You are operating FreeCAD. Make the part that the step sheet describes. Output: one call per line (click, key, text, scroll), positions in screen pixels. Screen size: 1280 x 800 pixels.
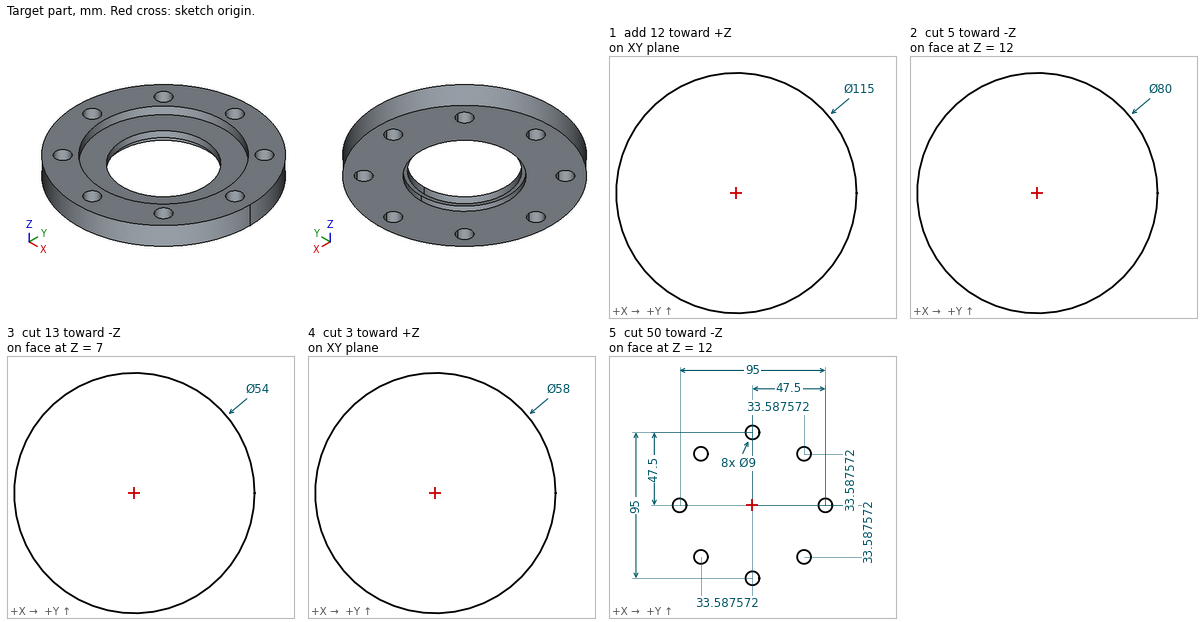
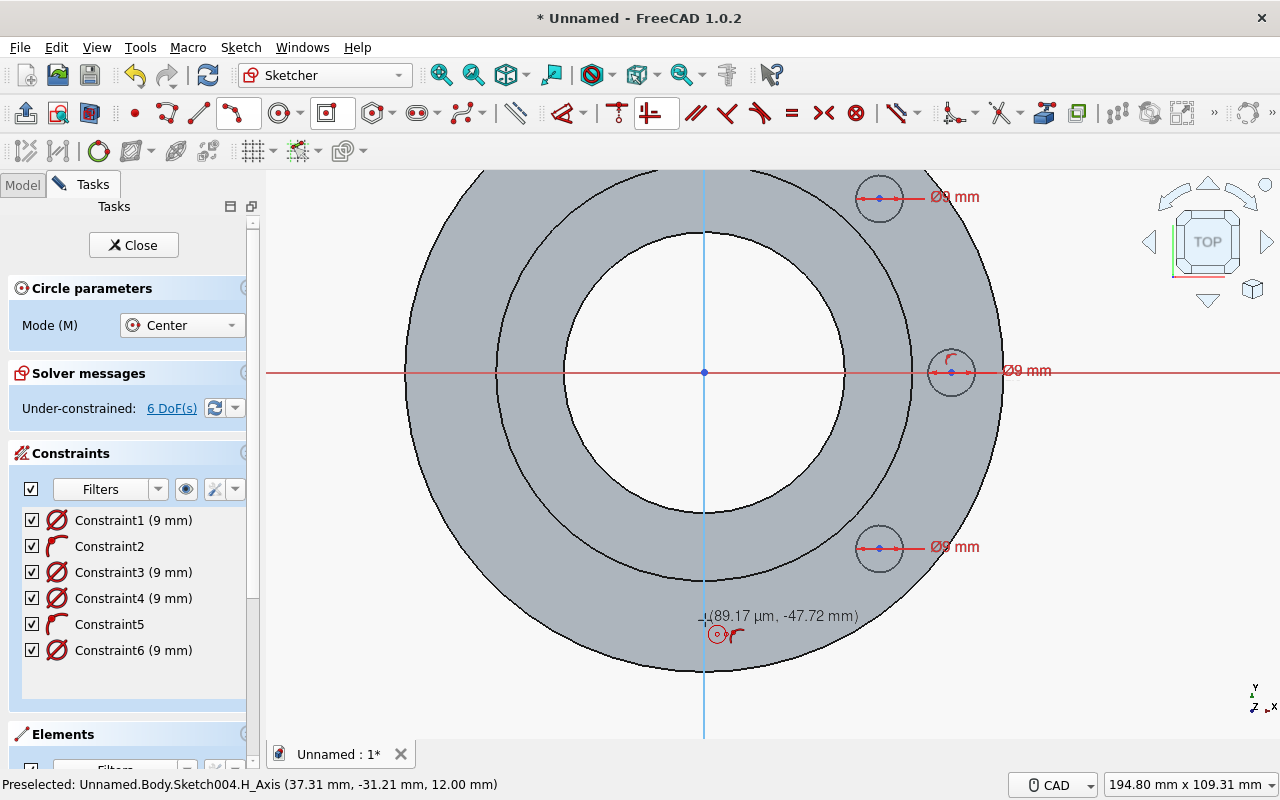
click(704, 620)
move(721, 603)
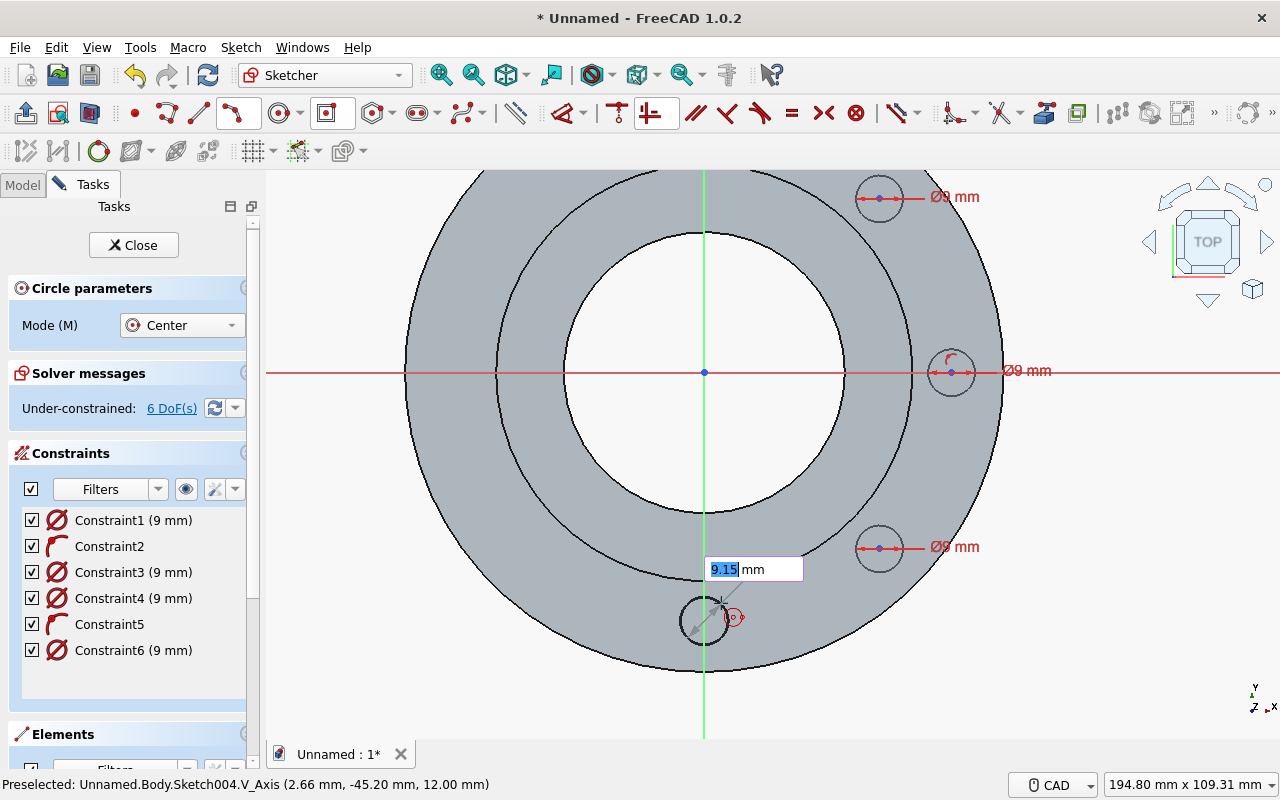
text(9)
key(Return)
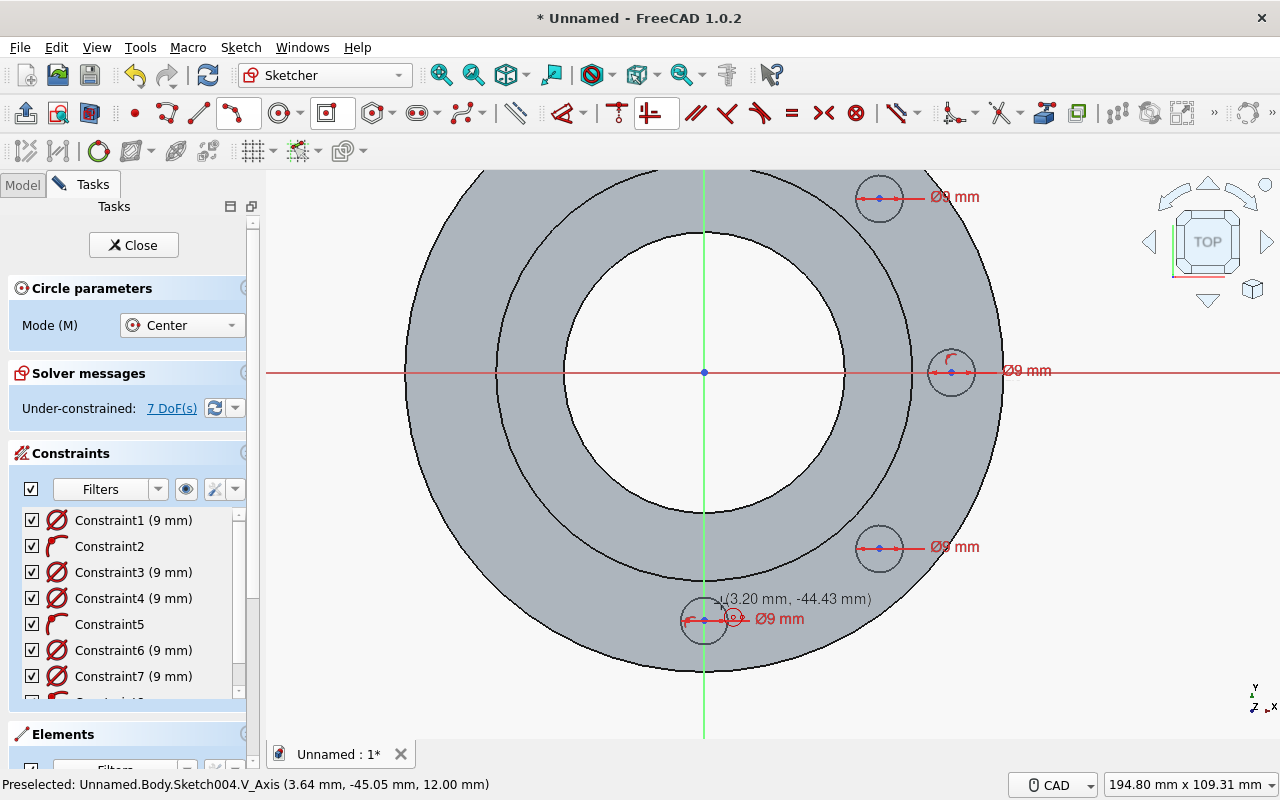
click(529, 548)
move(546, 531)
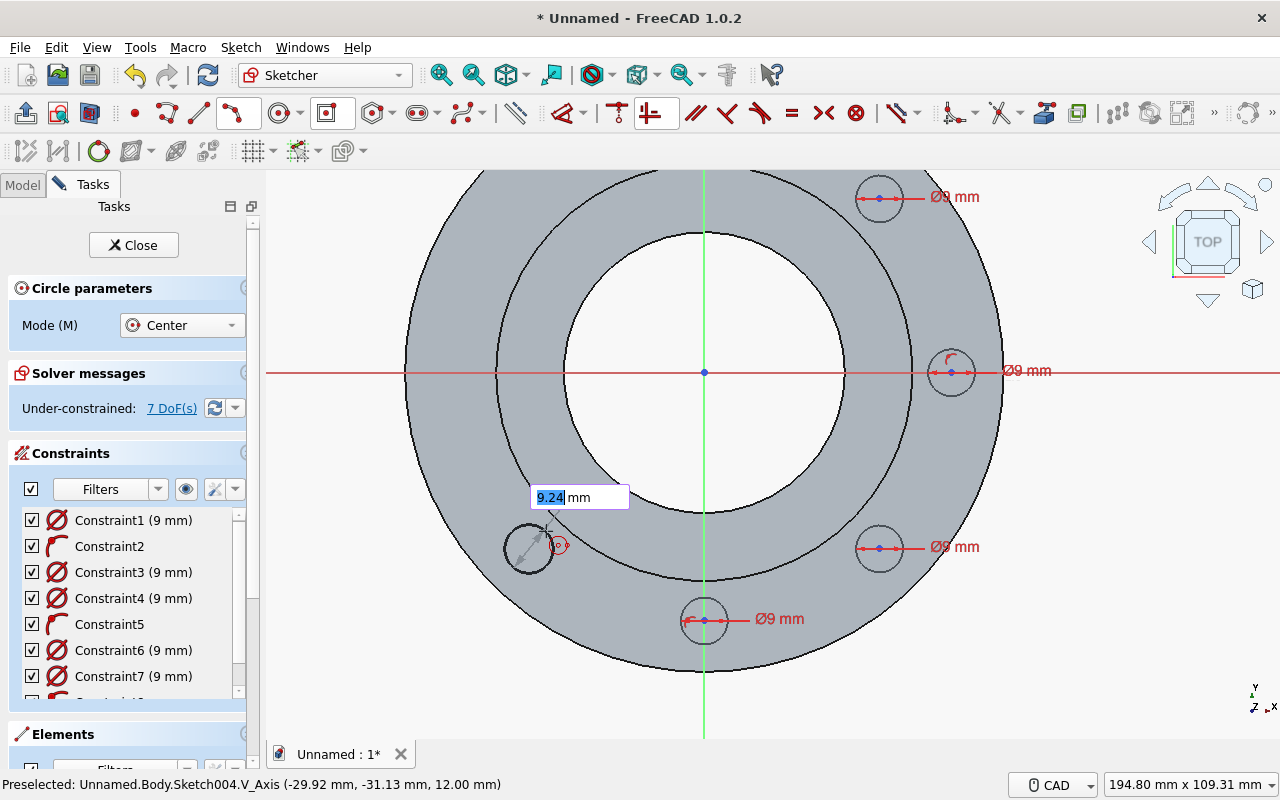
text(9)
key(Return)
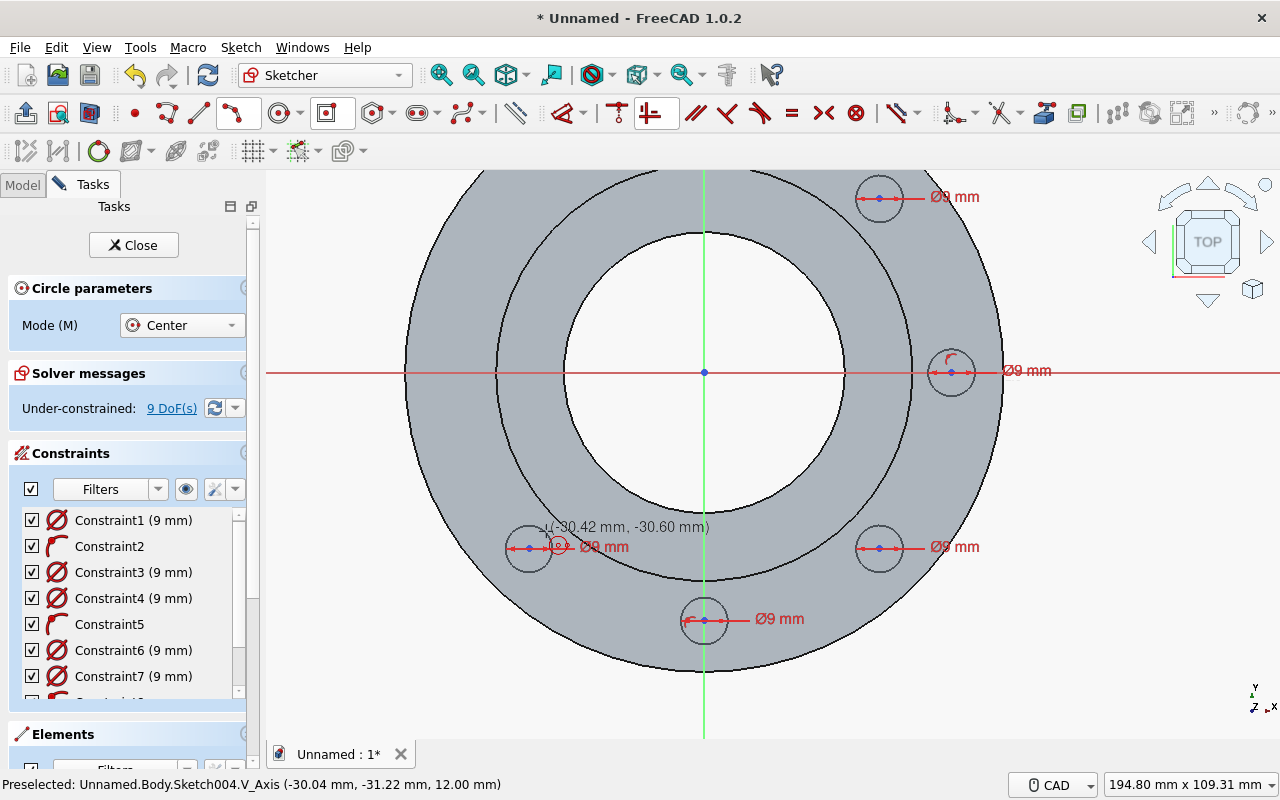
click(457, 373)
move(474, 356)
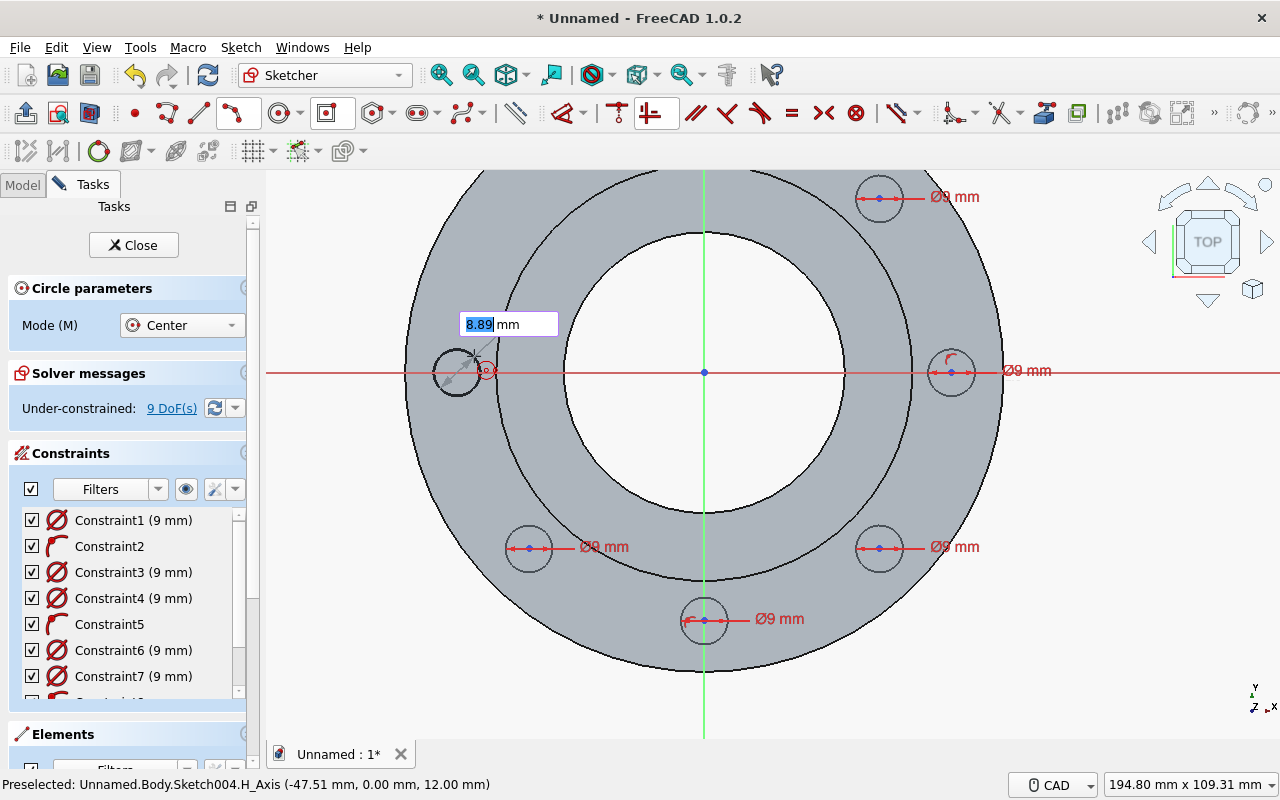
text(9)
key(Return)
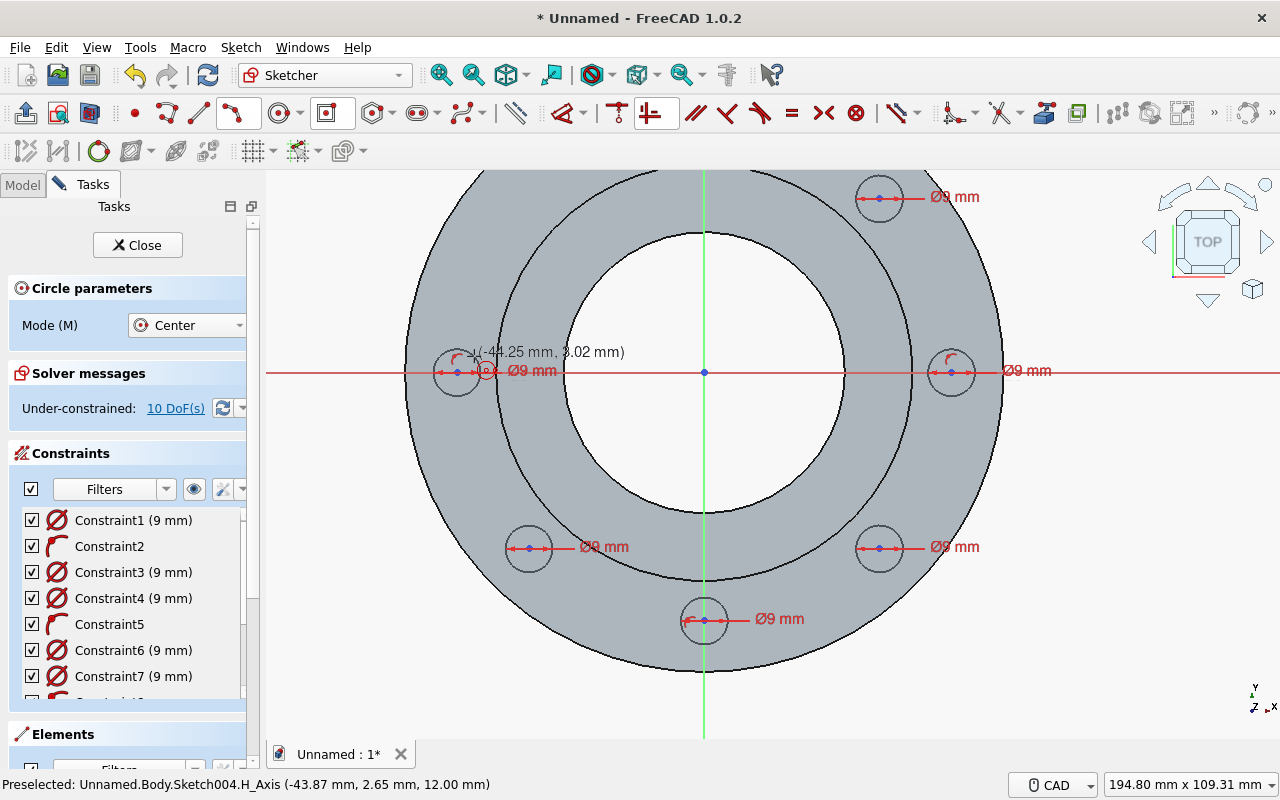
scroll(705, 621, down, 2)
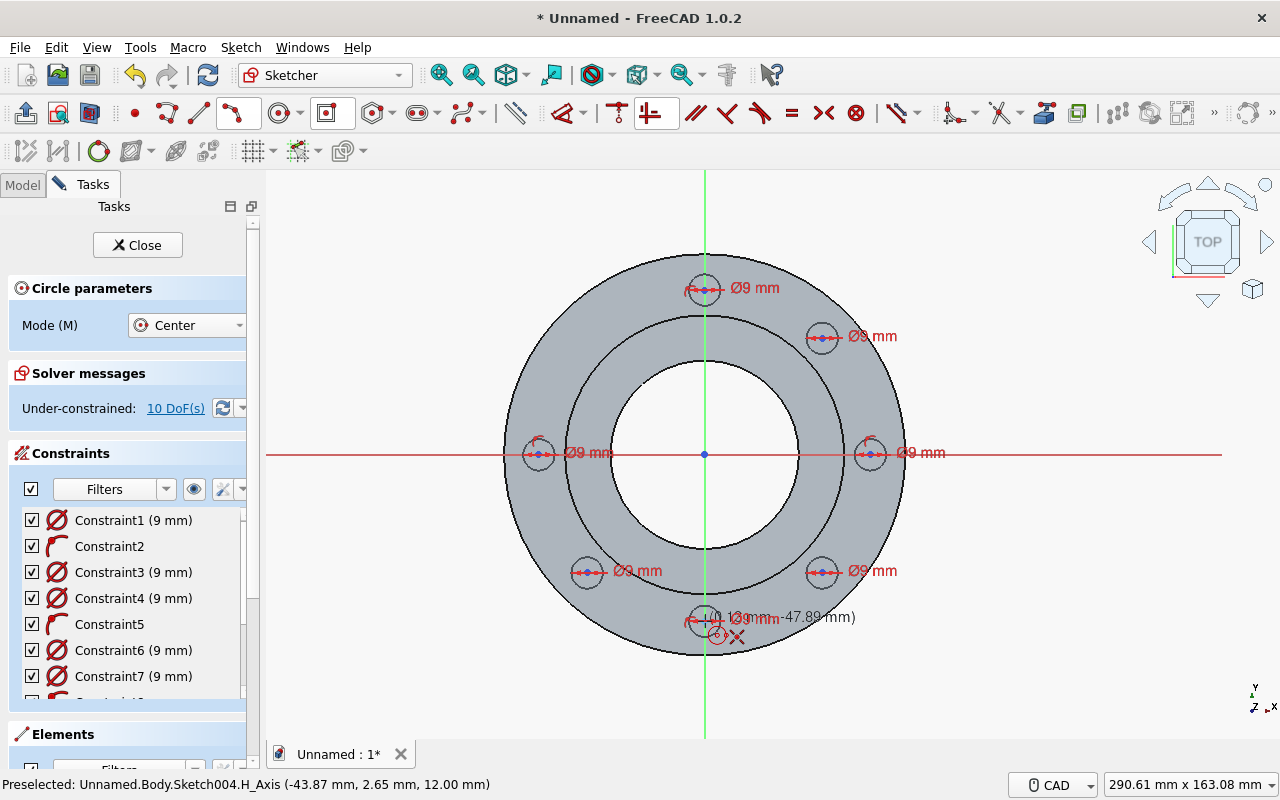
scroll(587, 338, up, 2)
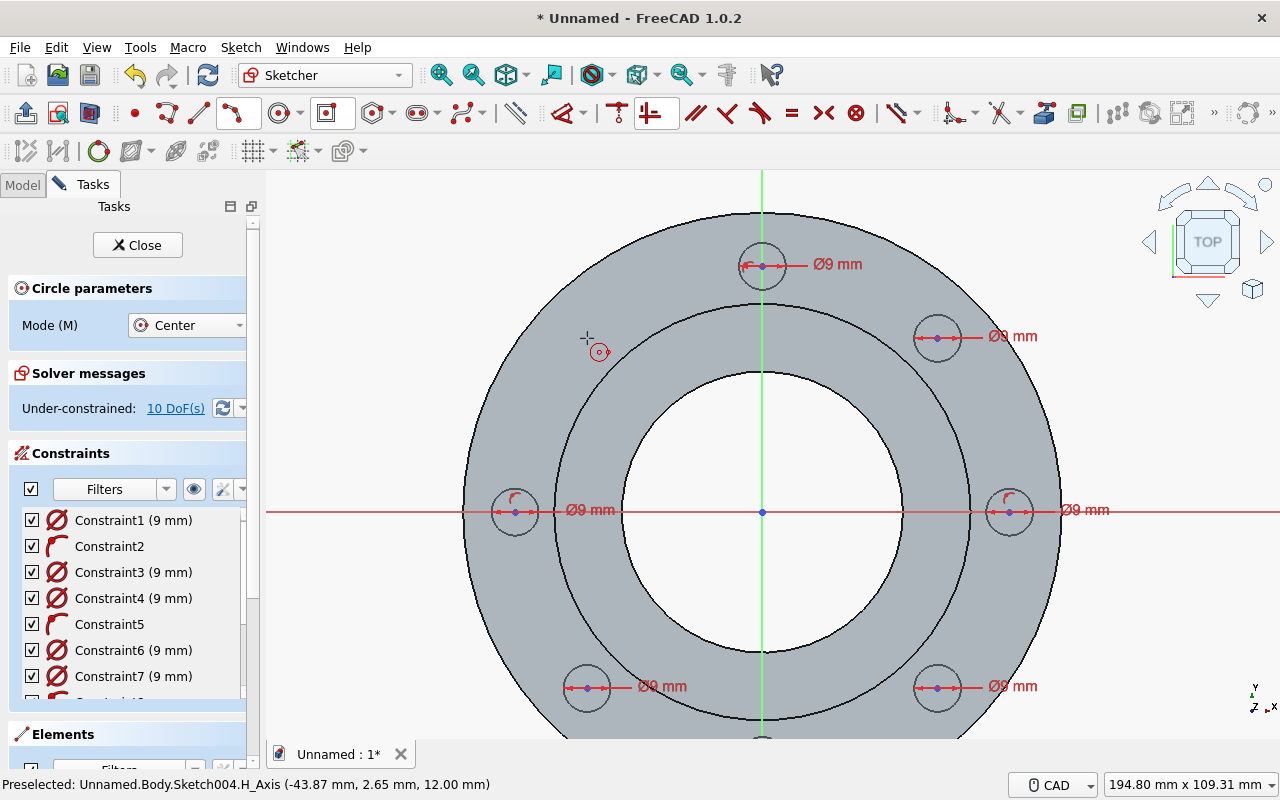
click(588, 337)
move(604, 321)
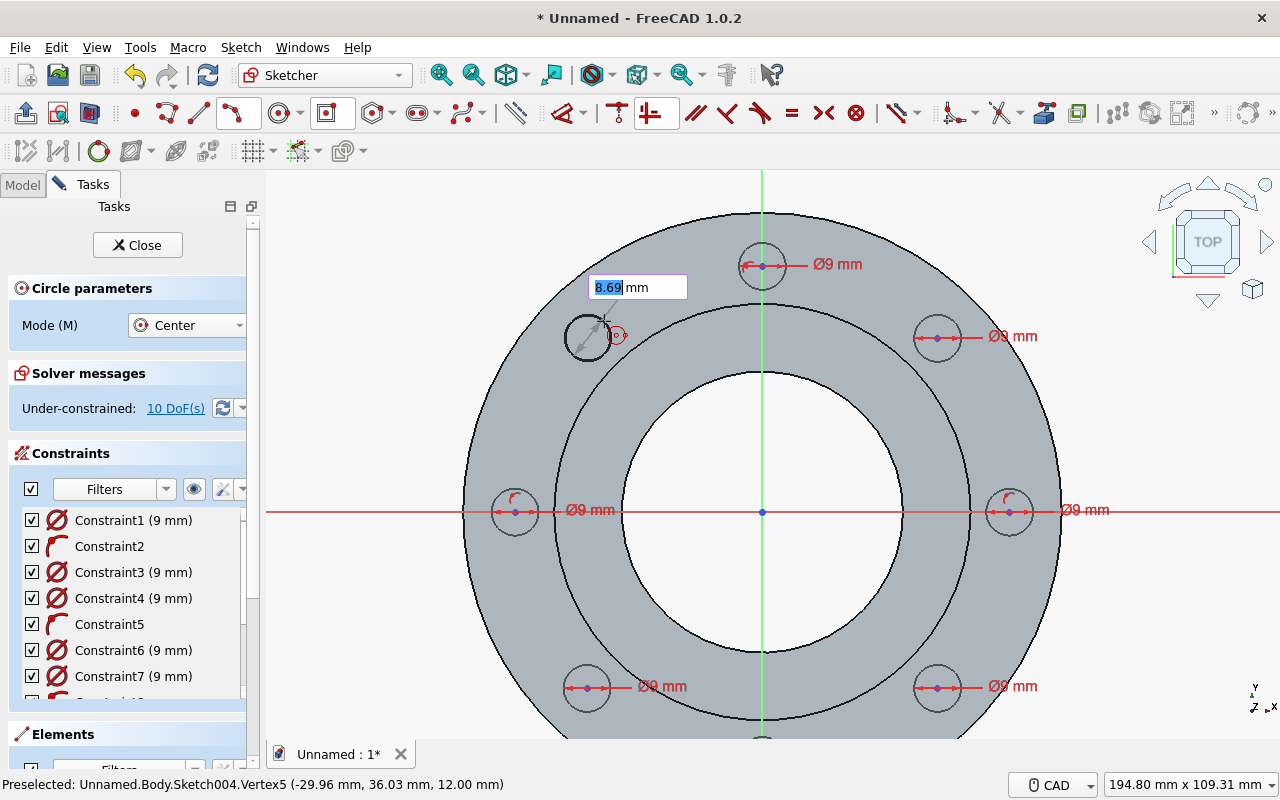
text(9)
key(Return)
key(Escape)